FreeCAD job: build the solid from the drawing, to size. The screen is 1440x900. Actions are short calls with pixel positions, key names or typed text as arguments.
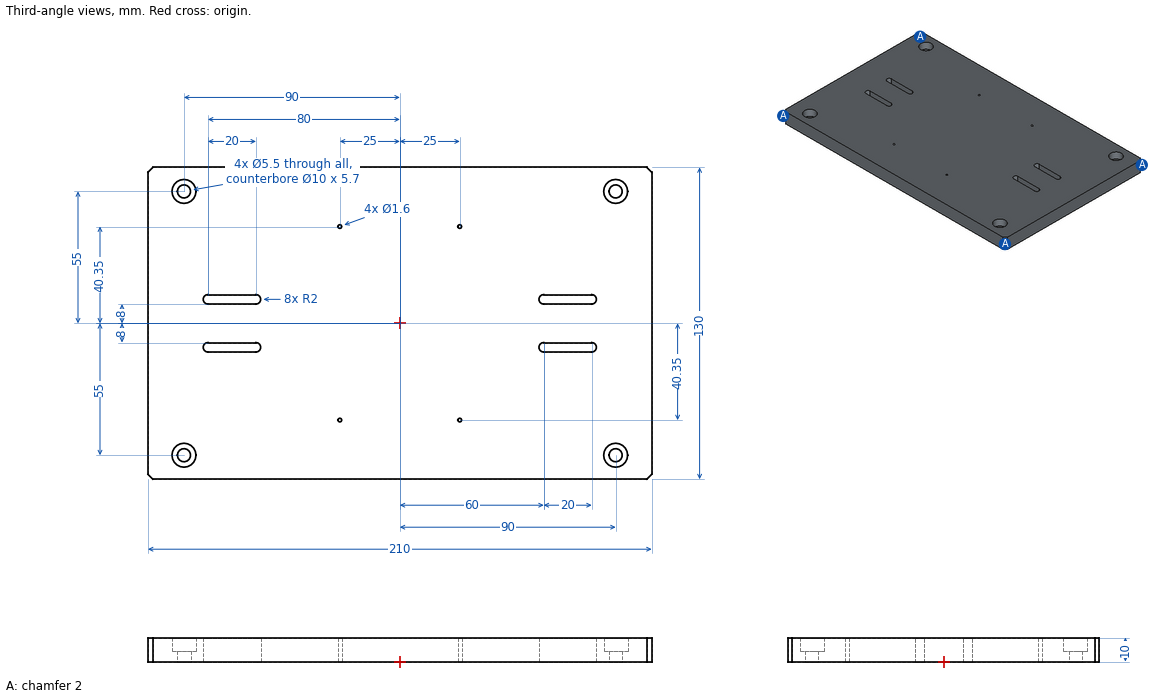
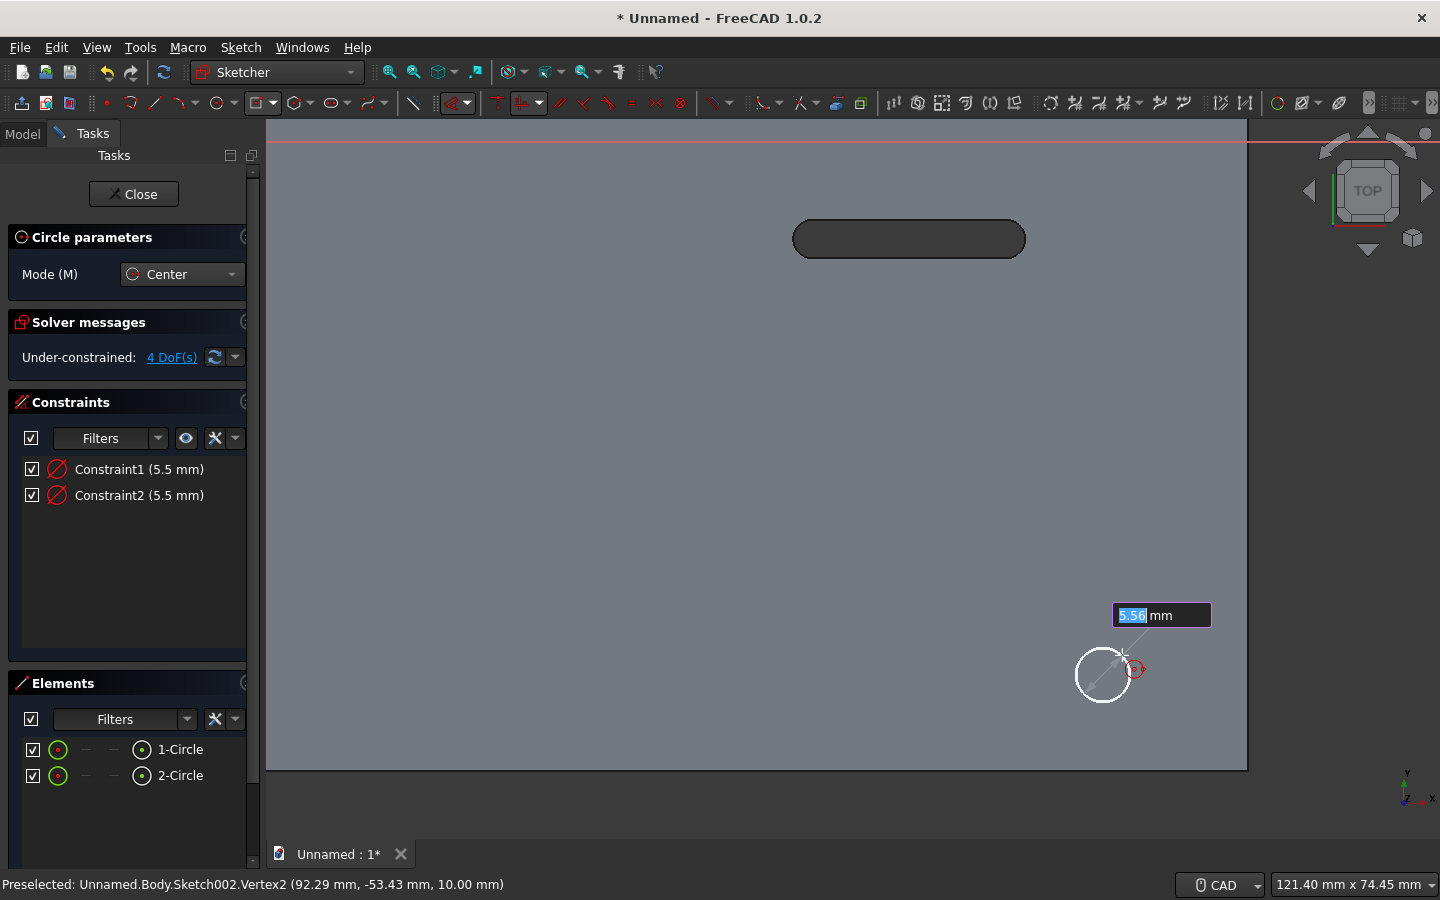
text(5.5)
key(Return)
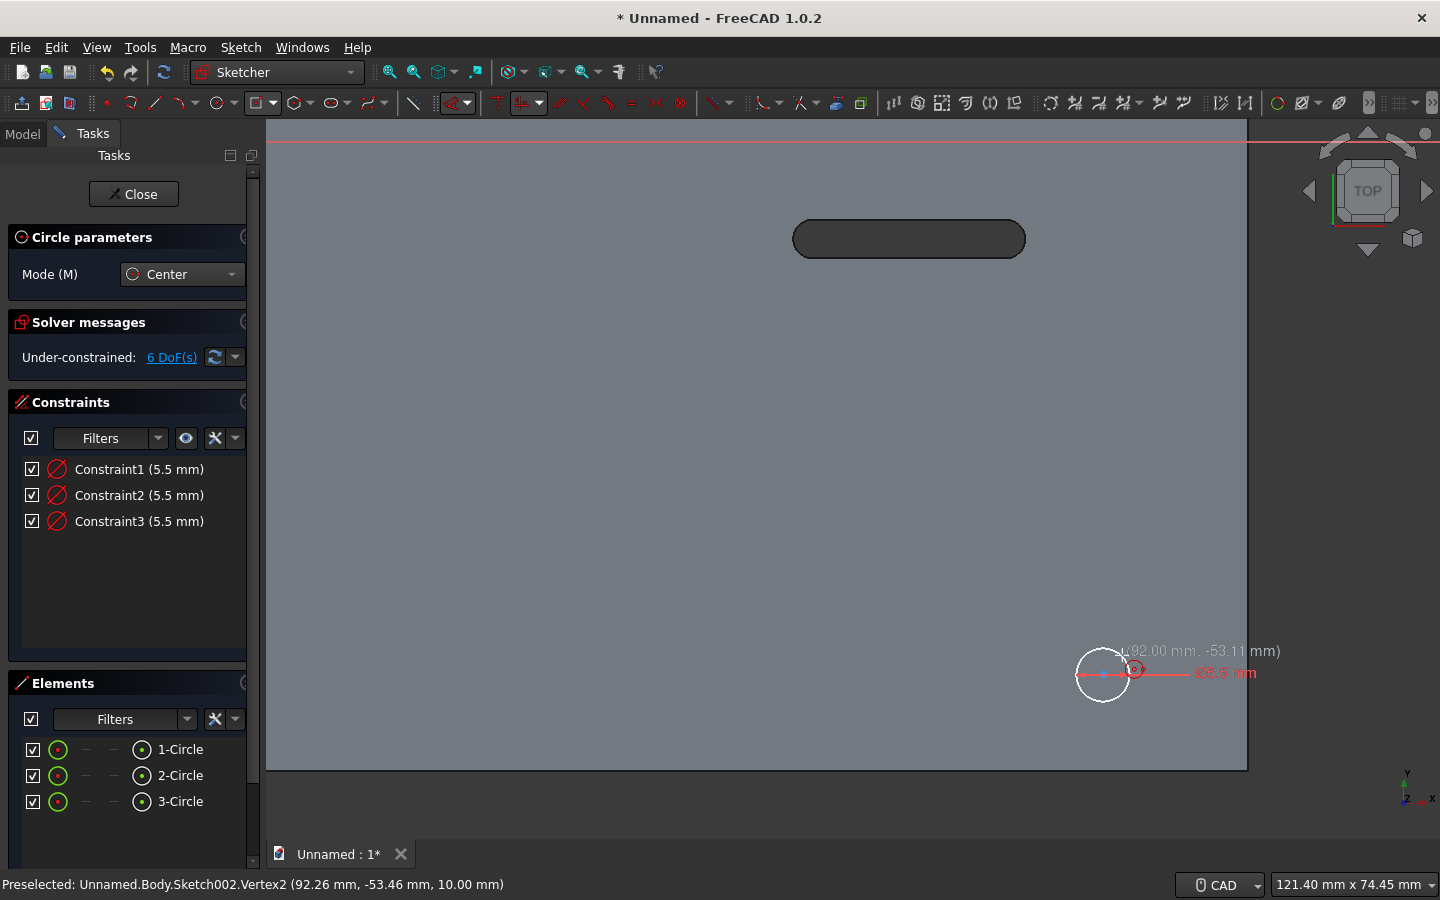
scroll(1106, 675, down, 5)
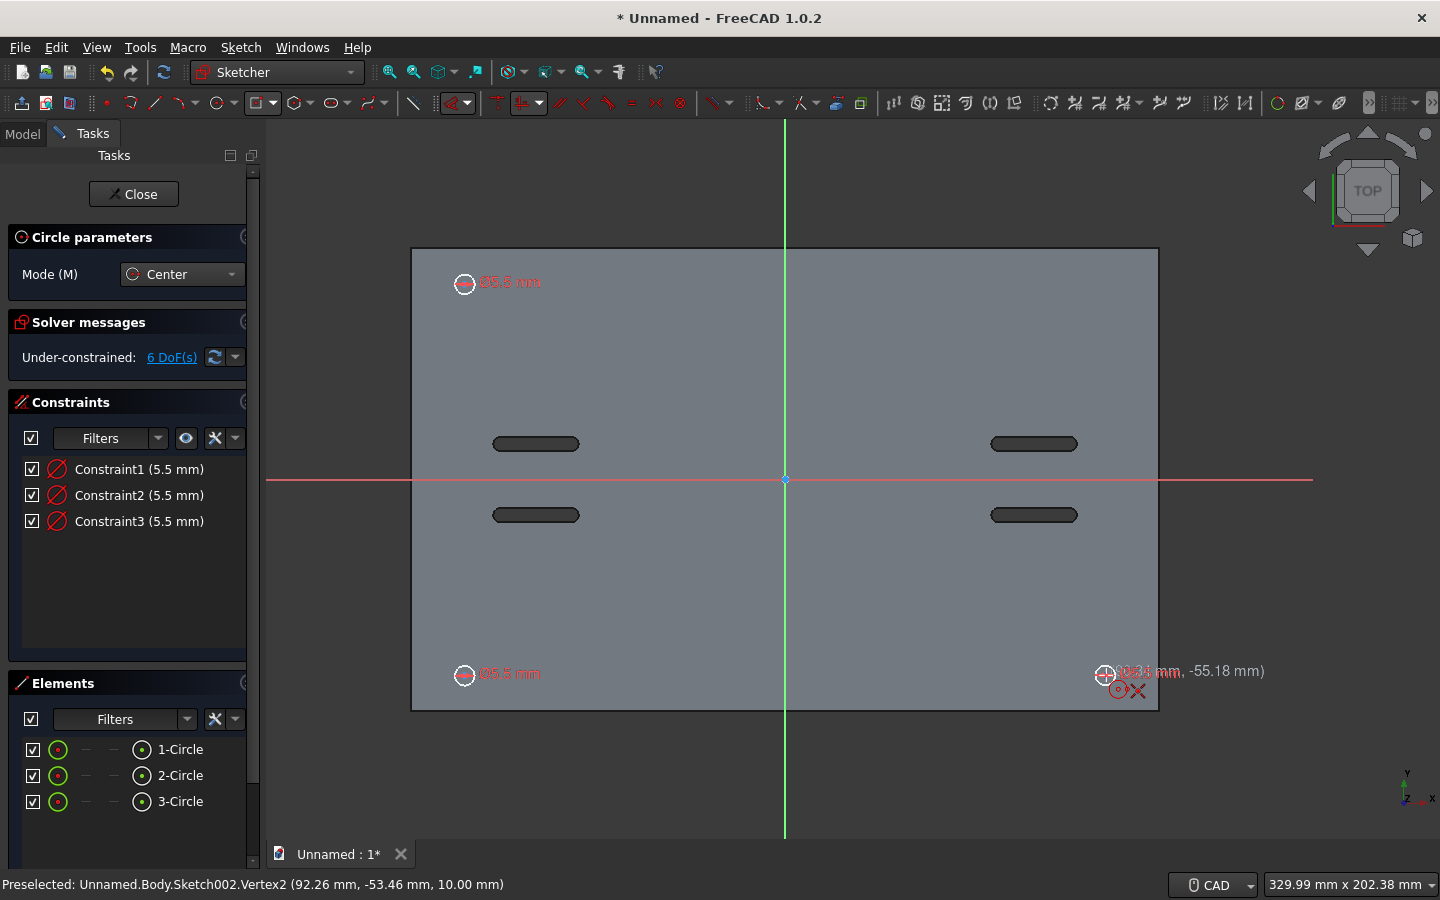
scroll(1105, 284, up, 5)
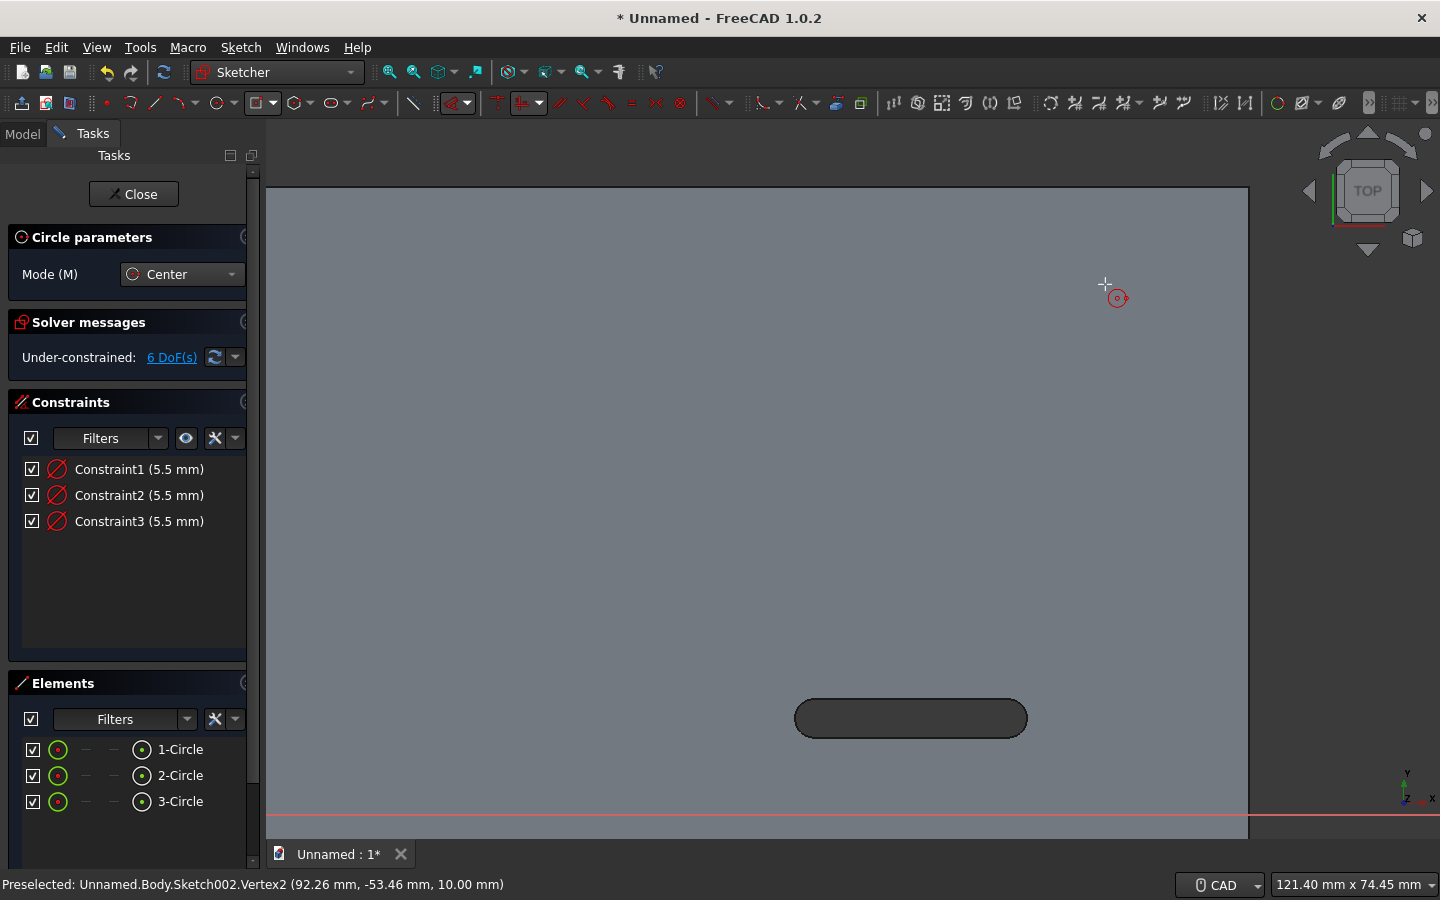
click(1104, 283)
move(1123, 264)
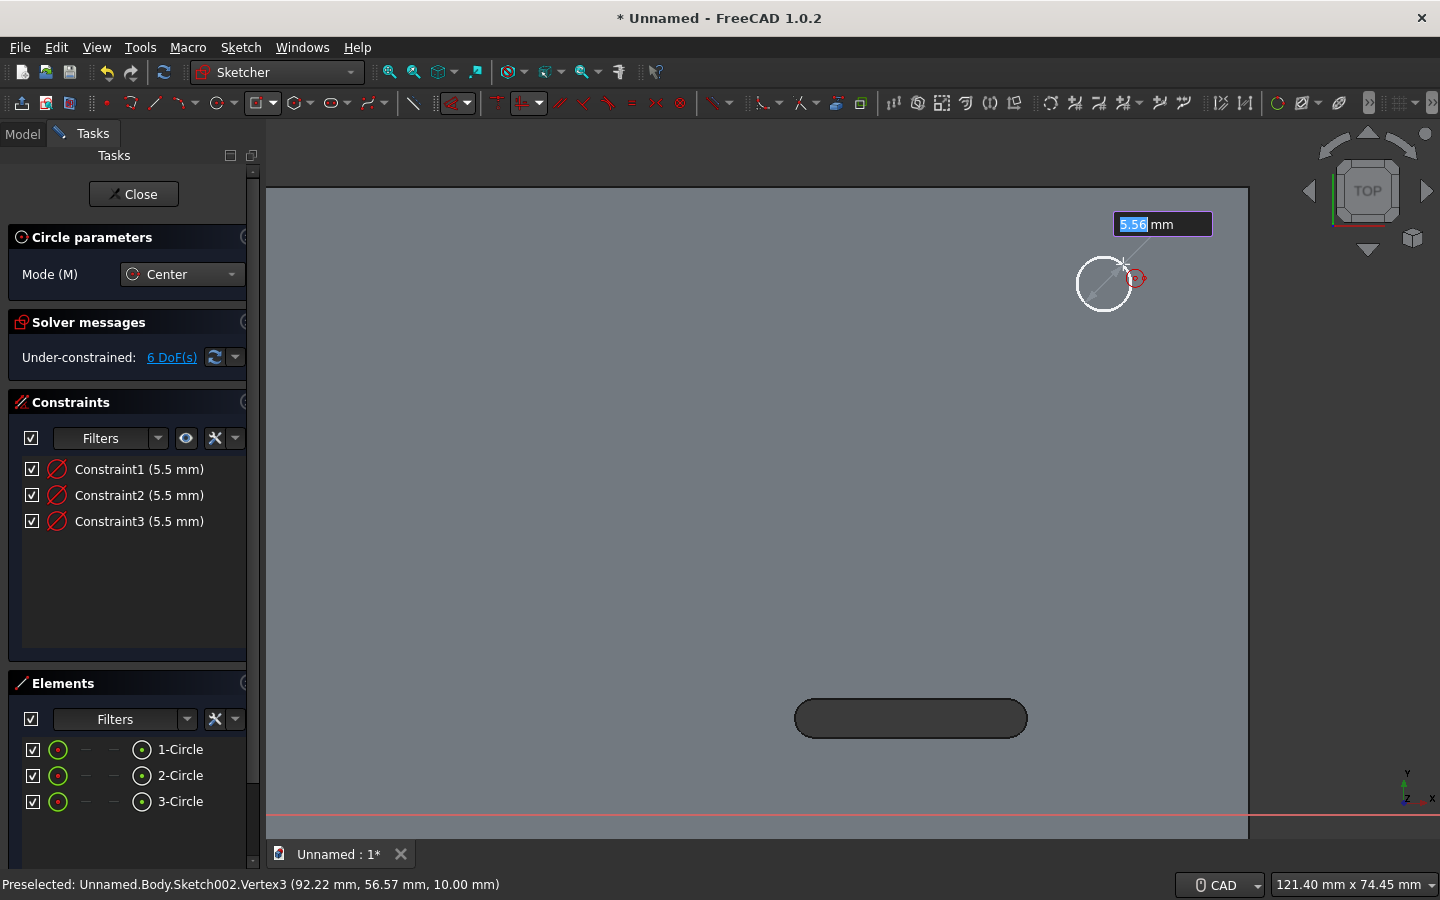
text(5.5)
key(Return)
key(Escape)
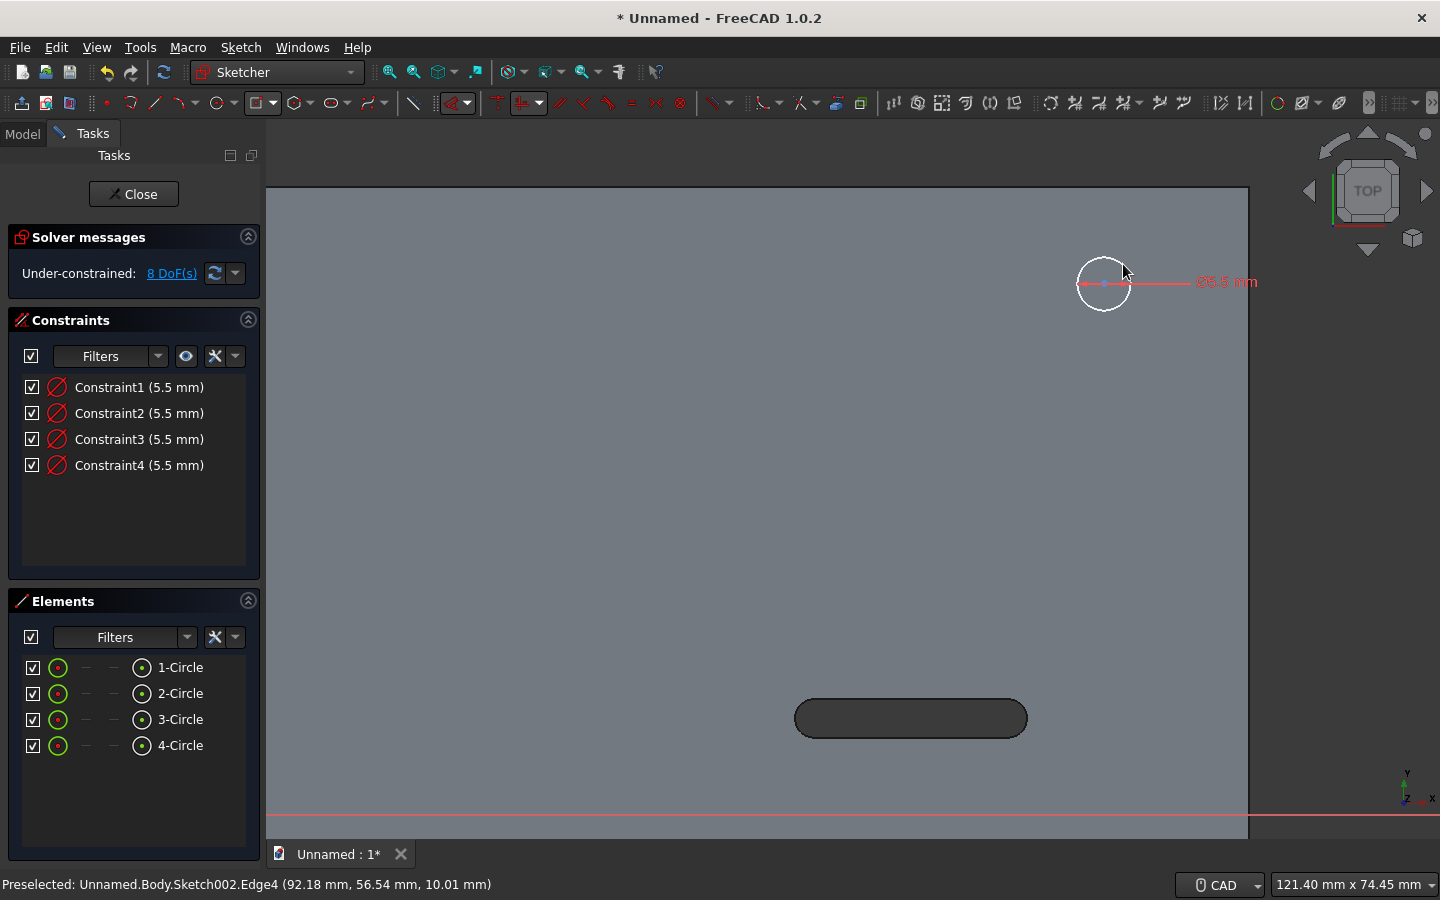
scroll(1105, 283, down, 5)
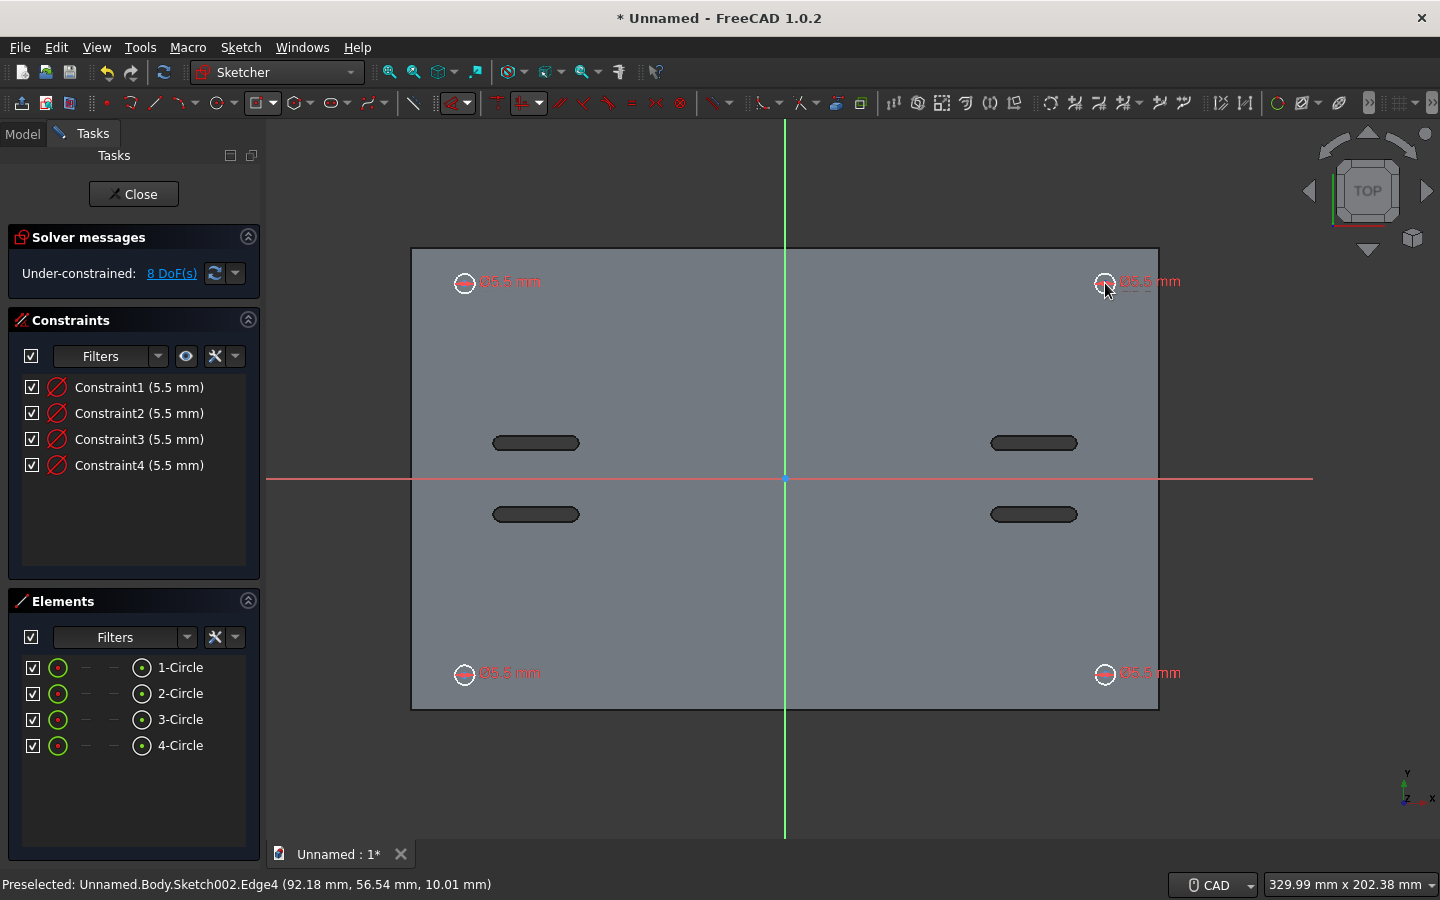
click(465, 284)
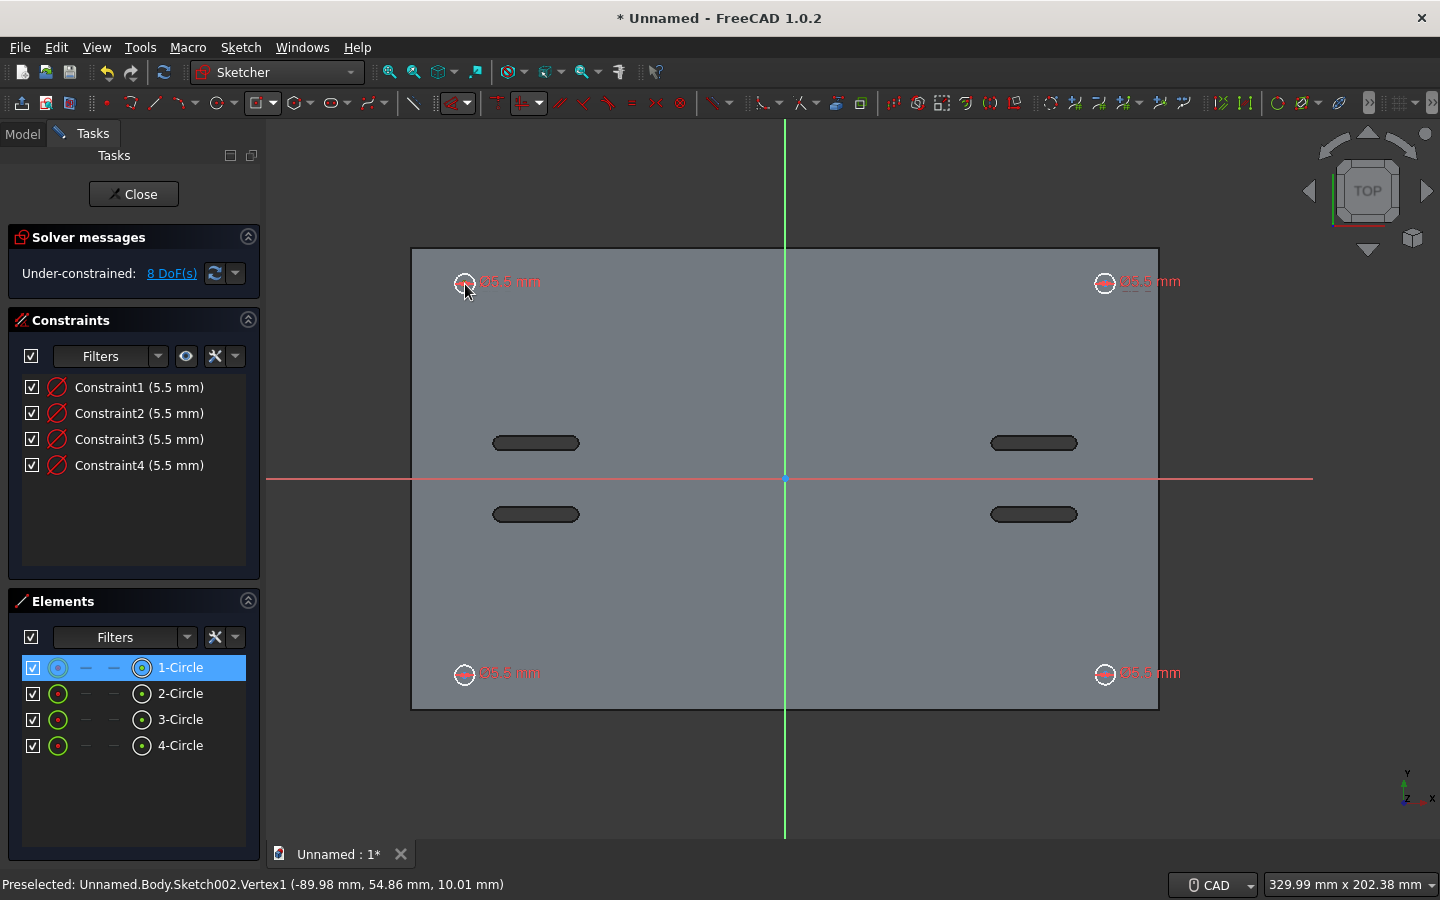
click(465, 675)